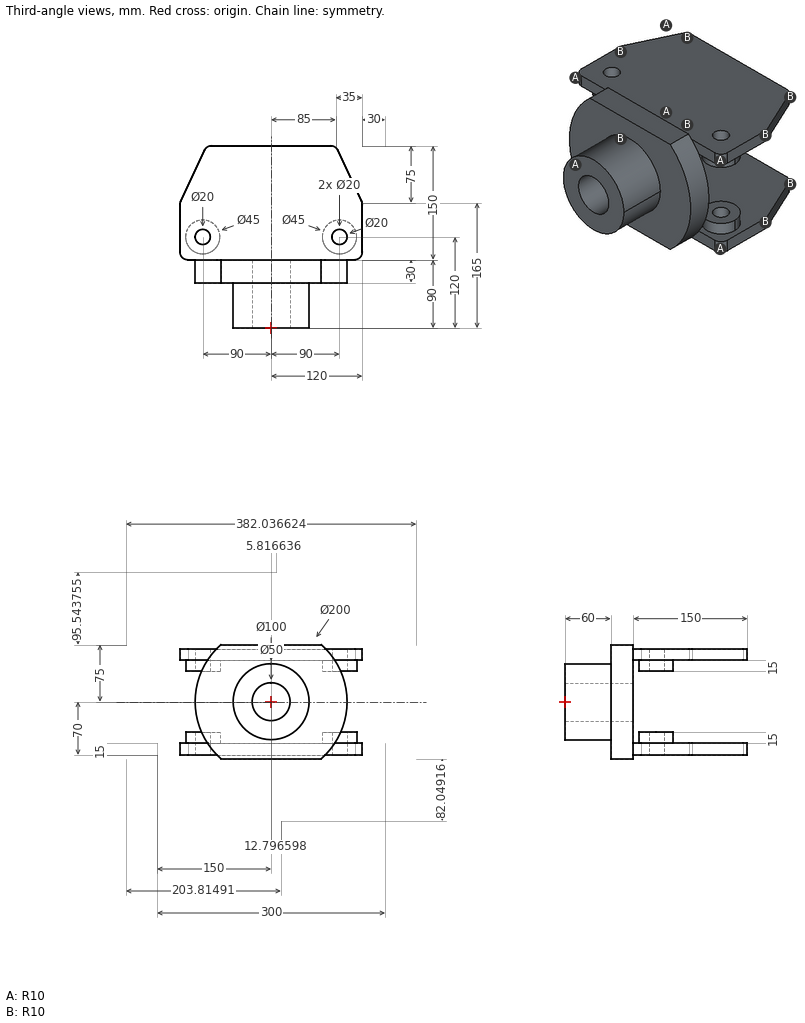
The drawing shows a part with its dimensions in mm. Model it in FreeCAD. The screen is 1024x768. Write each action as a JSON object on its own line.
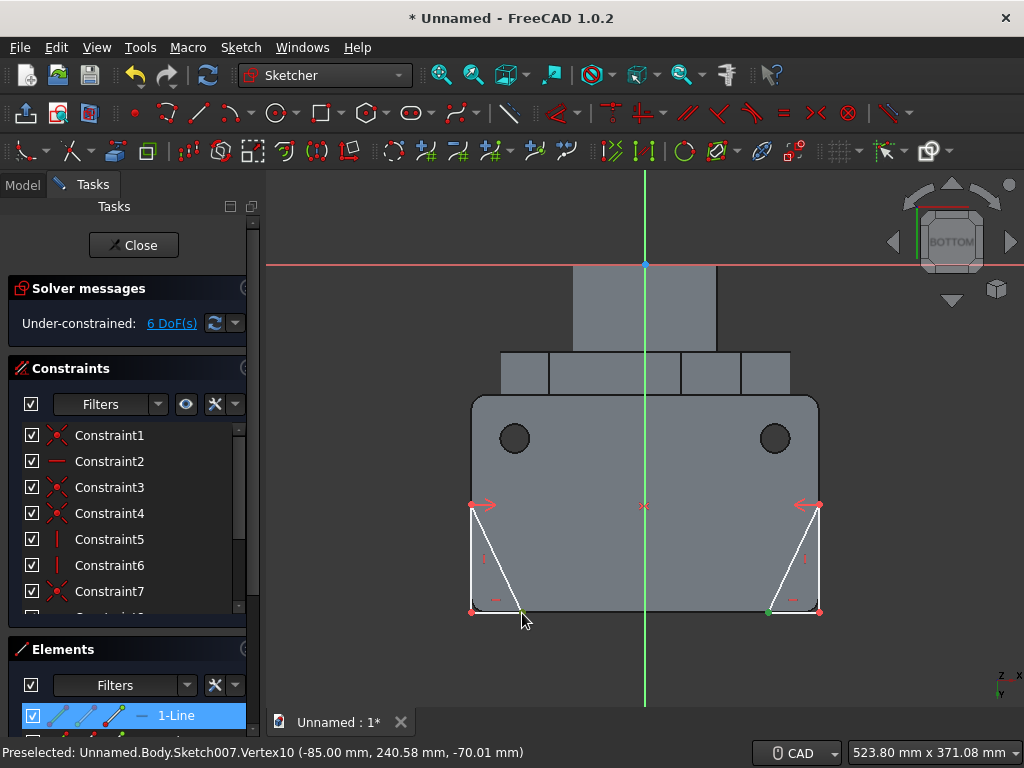
{"action": "left_click", "coordinate": [645, 645]}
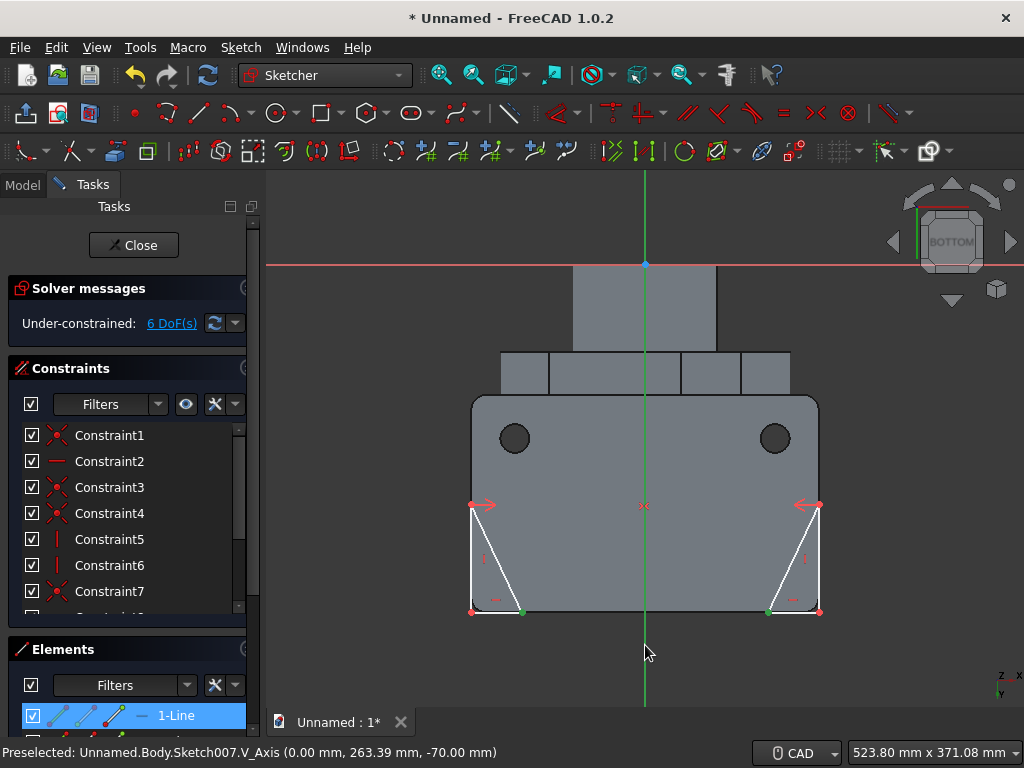
{"action": "left_click", "coordinate": [816, 114]}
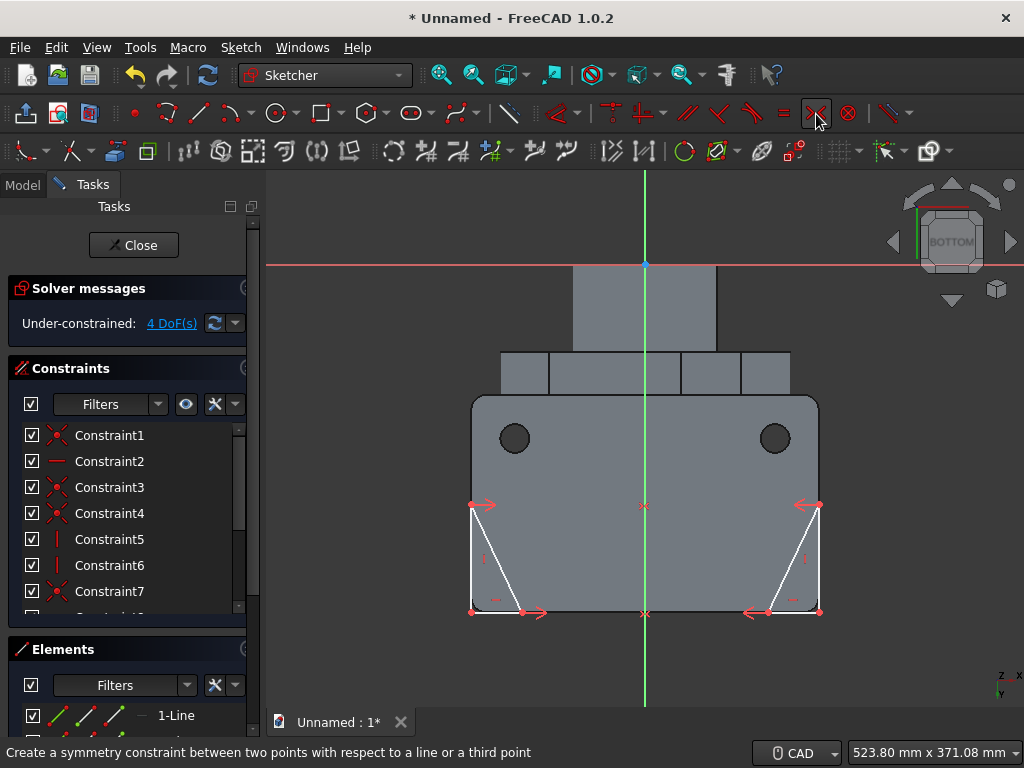
{"action": "key", "text": "d"}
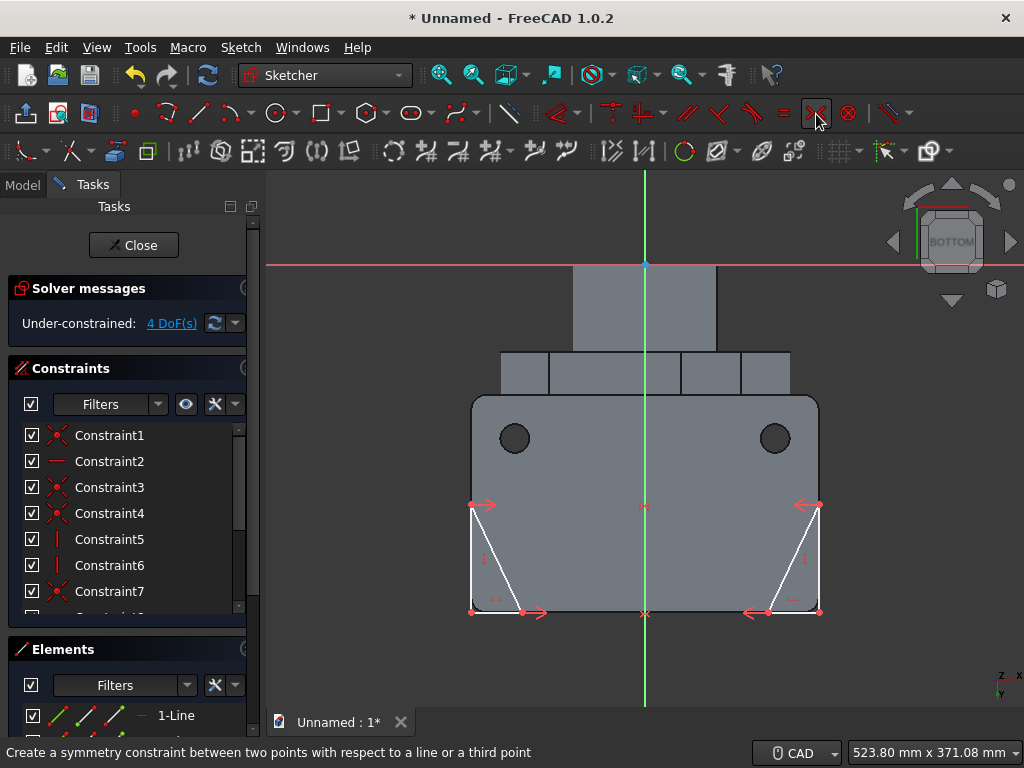
{"action": "left_click", "coordinate": [783, 613]}
{"action": "left_click", "coordinate": [793, 647]}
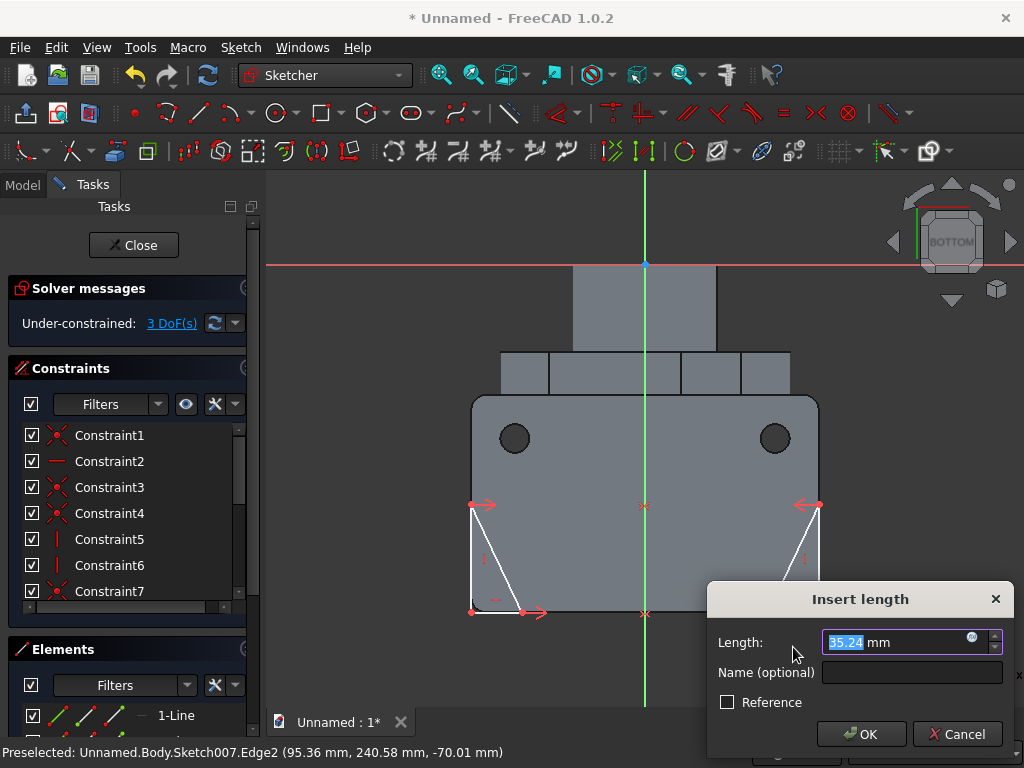
{"action": "type", "text": "35"}
{"action": "key", "text": "Return"}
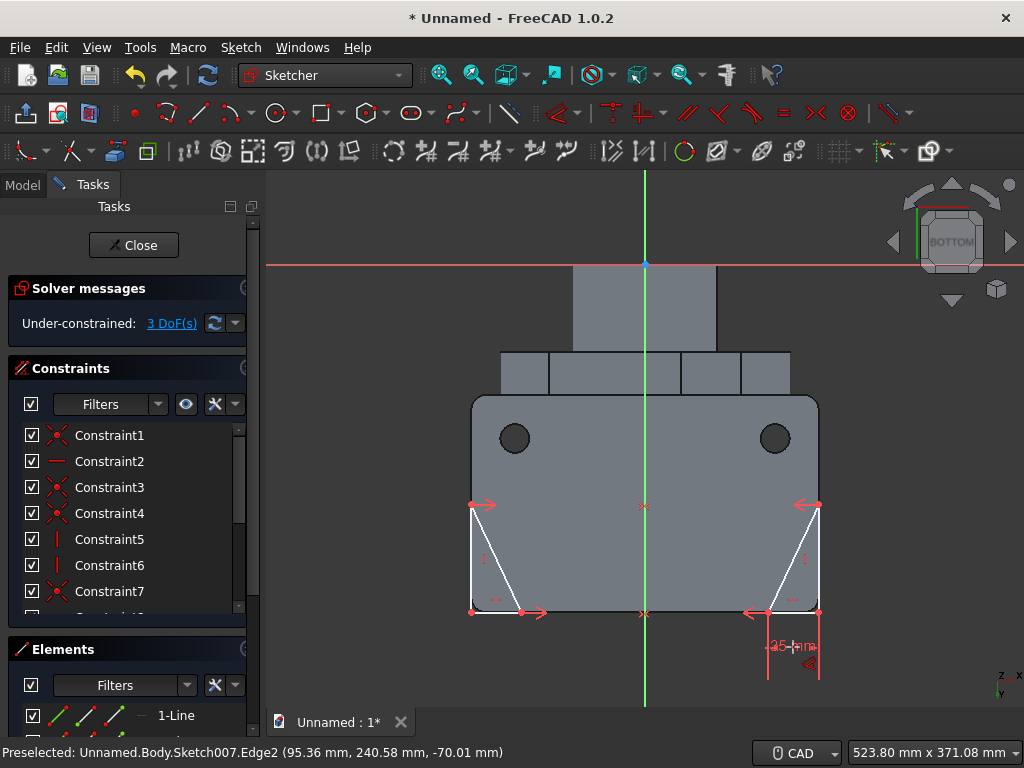
{"action": "left_click", "coordinate": [819, 581]}
{"action": "left_click", "coordinate": [853, 559]}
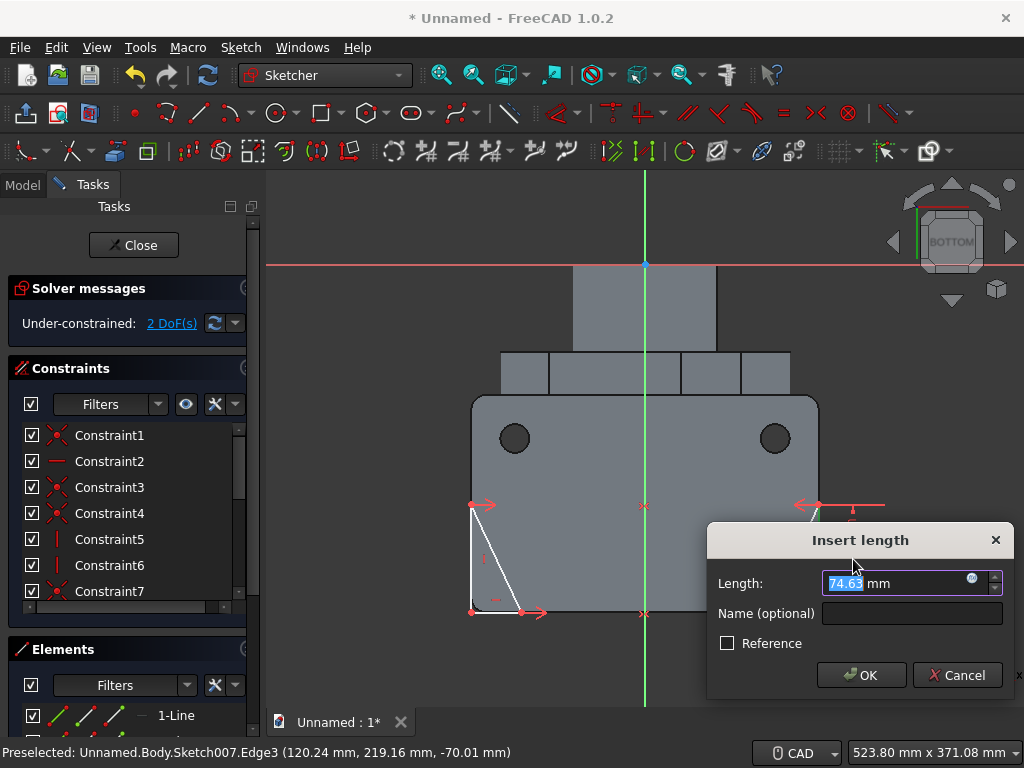
{"action": "type", "text": "75"}
{"action": "key", "text": "Return"}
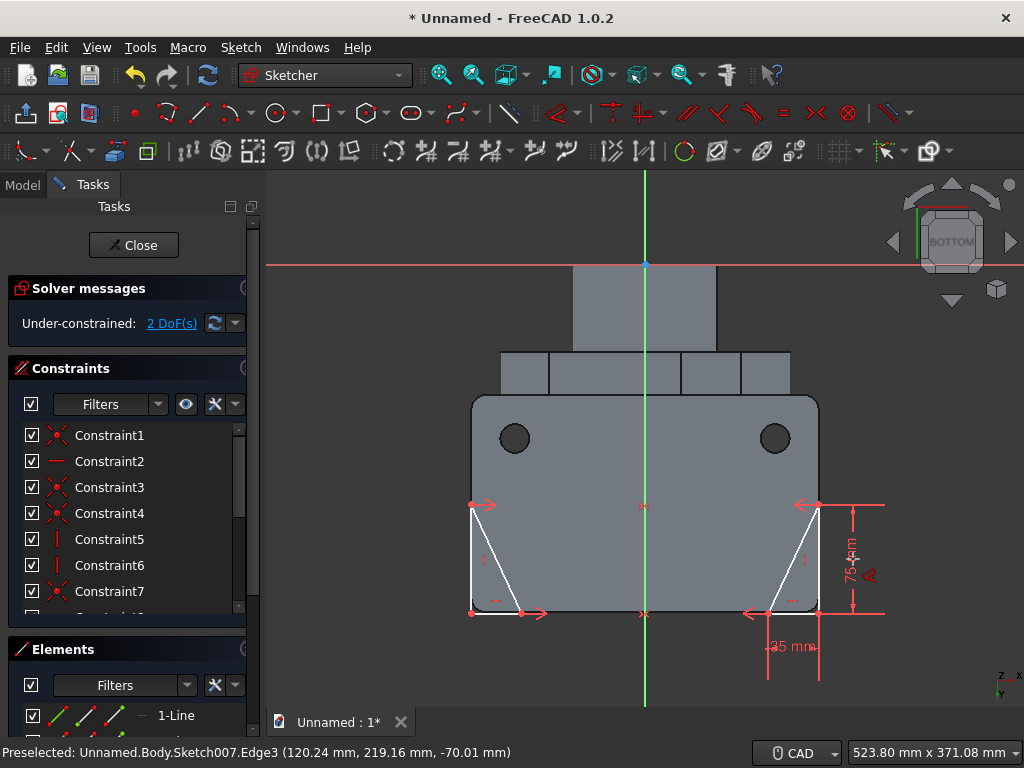
{"action": "left_click", "coordinate": [768, 614]}
{"action": "left_click", "coordinate": [707, 648]}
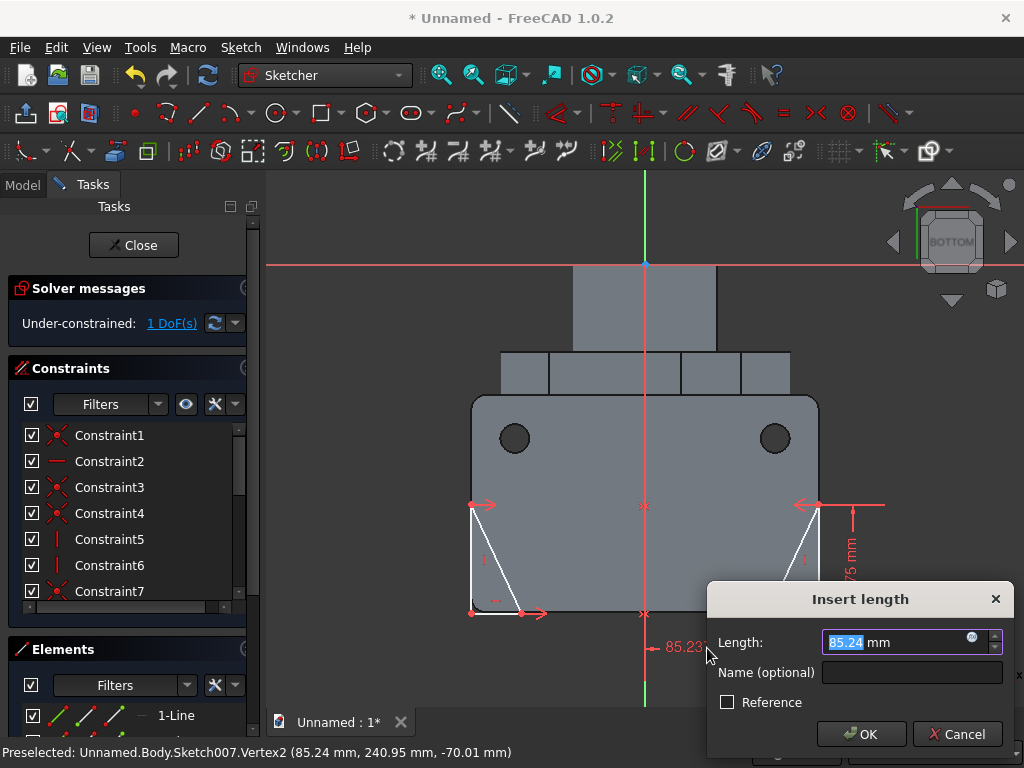
{"action": "type", "text": "85"}
{"action": "key", "text": "Return"}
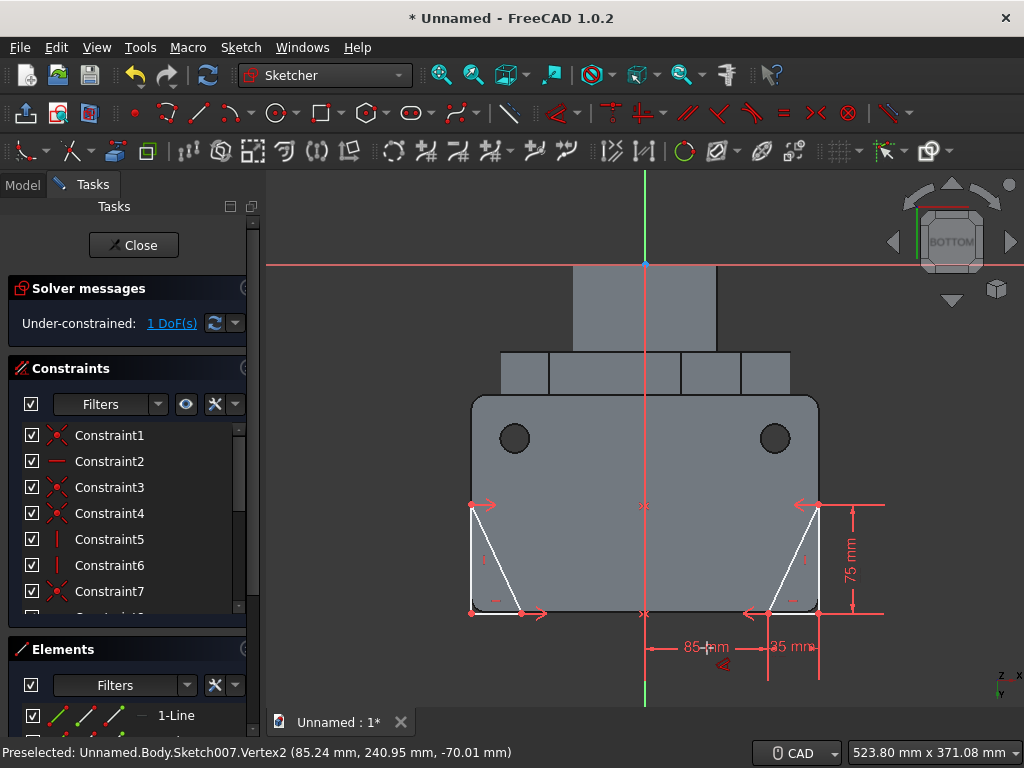
{"action": "left_click", "coordinate": [819, 505]}
{"action": "left_click", "coordinate": [853, 385]}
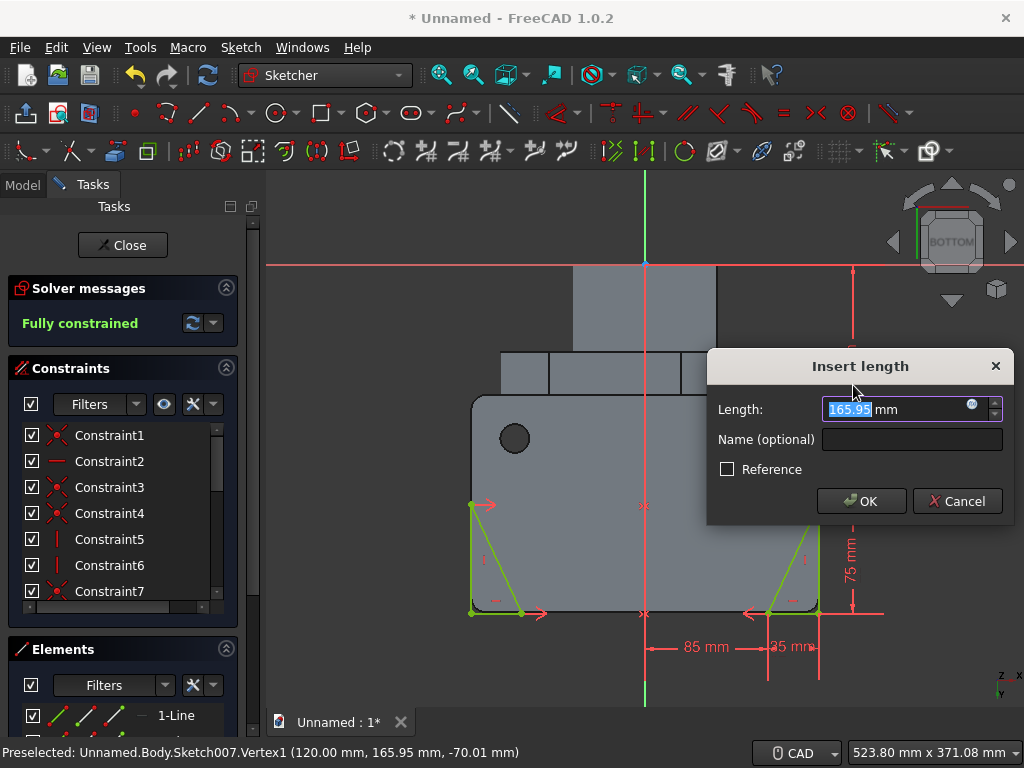
{"action": "type", "text": "165"}
{"action": "key", "text": "Return"}
{"action": "key", "text": "Escape"}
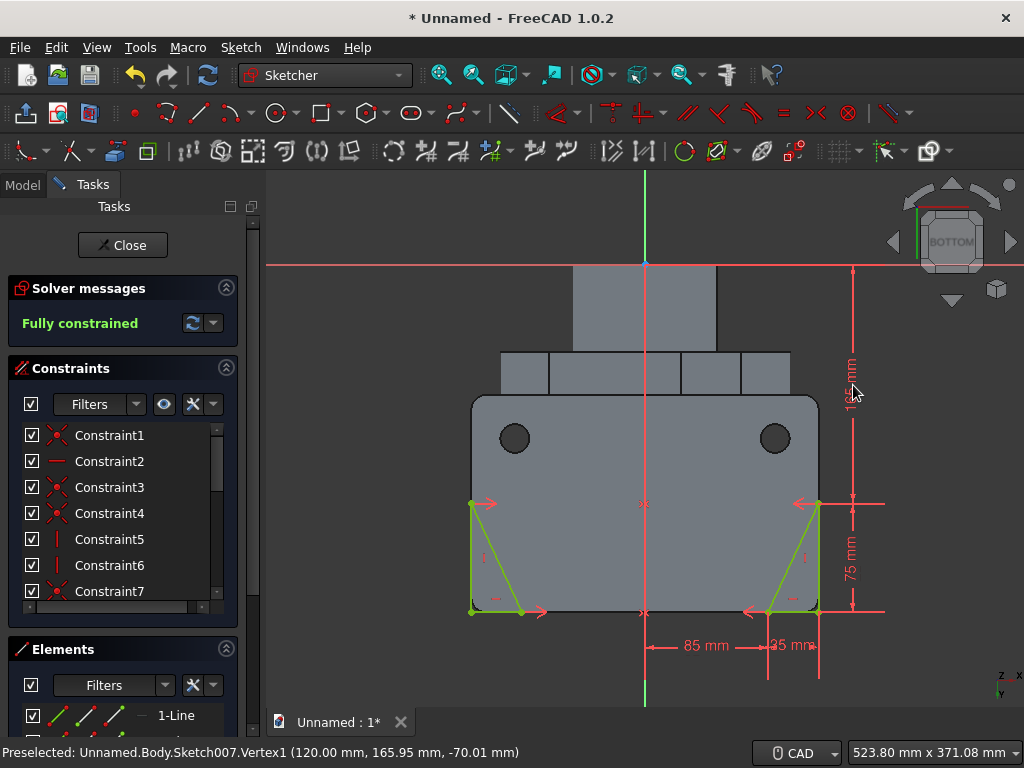
{"action": "left_click", "coordinate": [123, 245]}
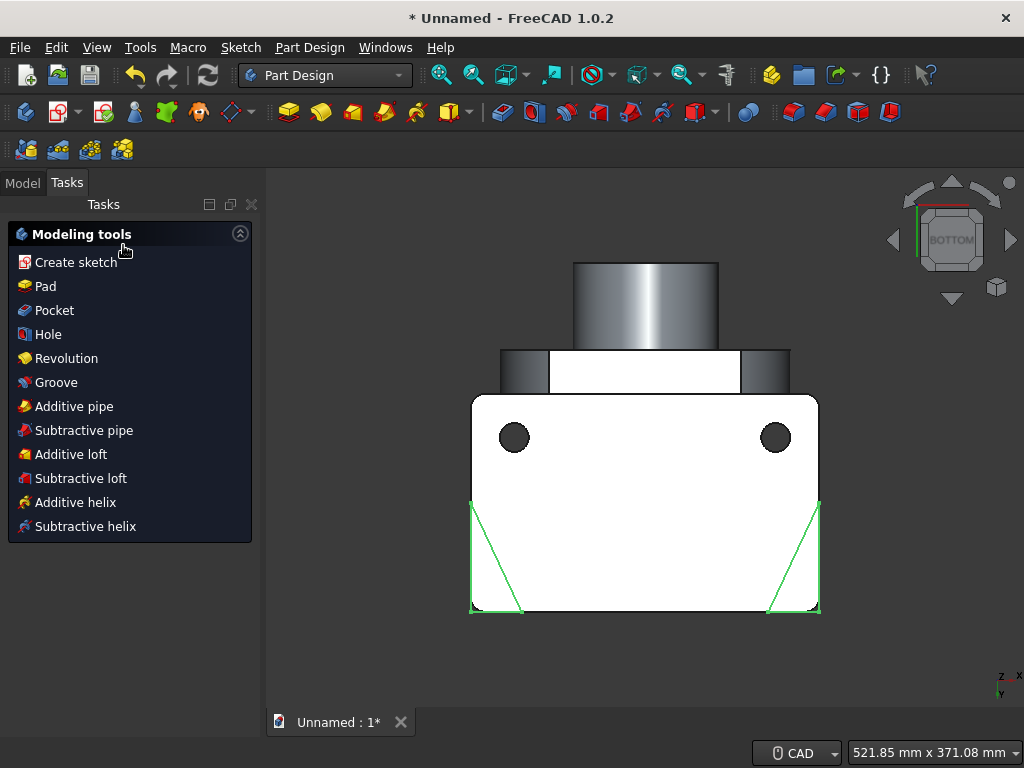
{"action": "left_click", "coordinate": [504, 112]}